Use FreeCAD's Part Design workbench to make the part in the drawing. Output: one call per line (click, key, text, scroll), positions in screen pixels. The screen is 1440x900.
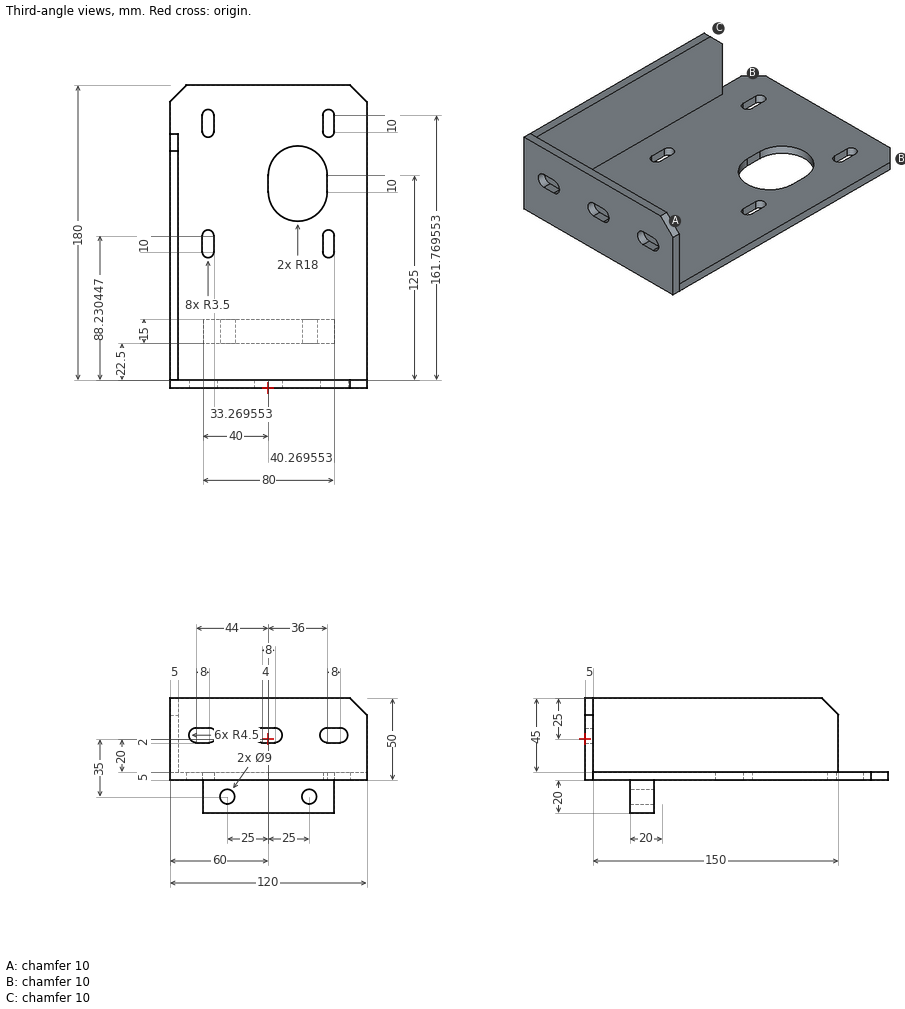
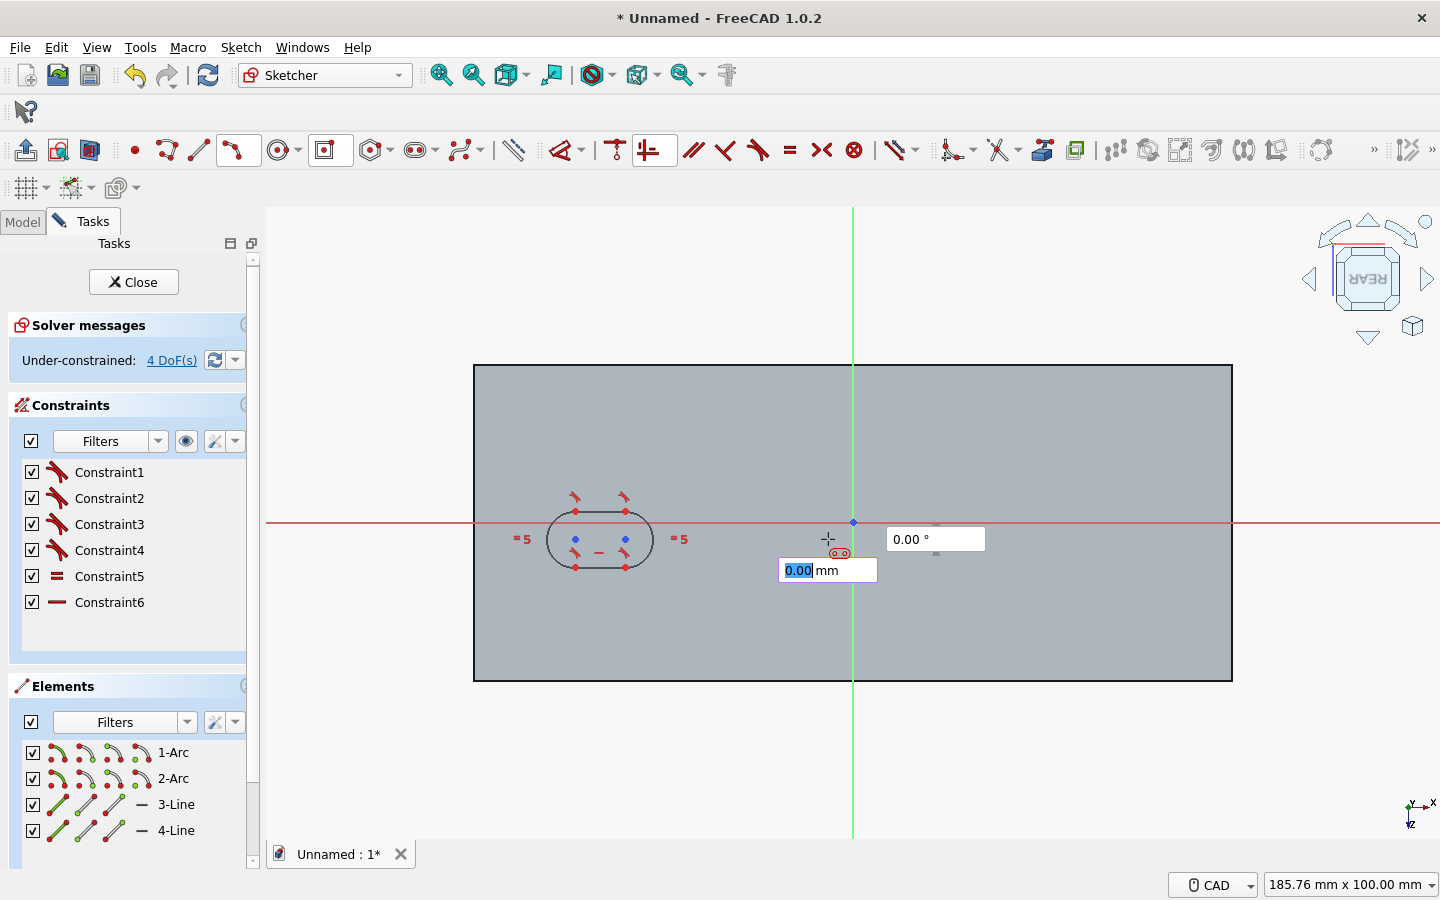
click(878, 539)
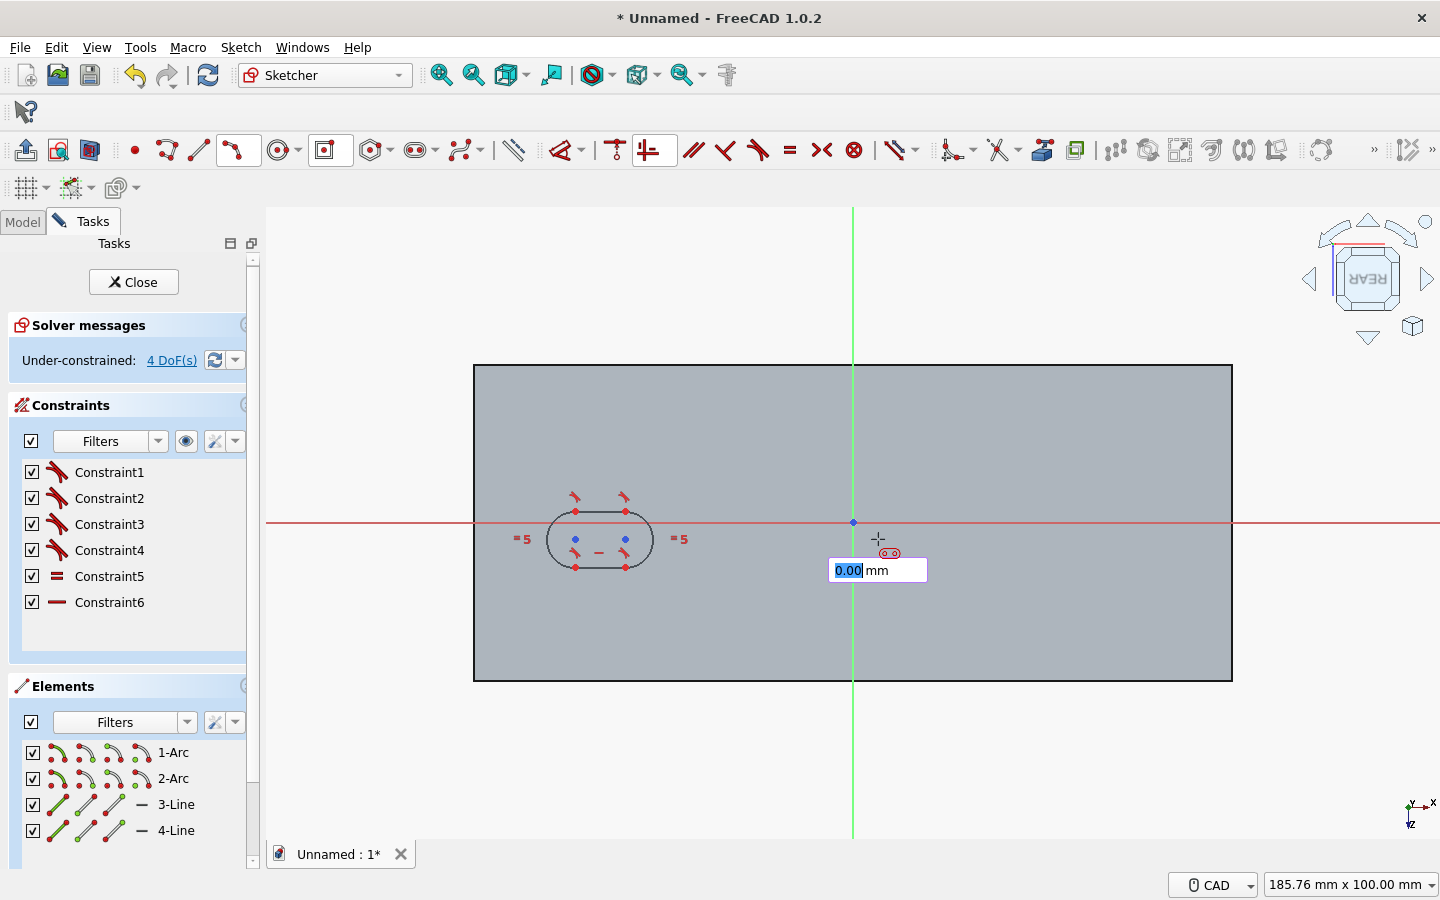
scroll(861, 510, up, 4)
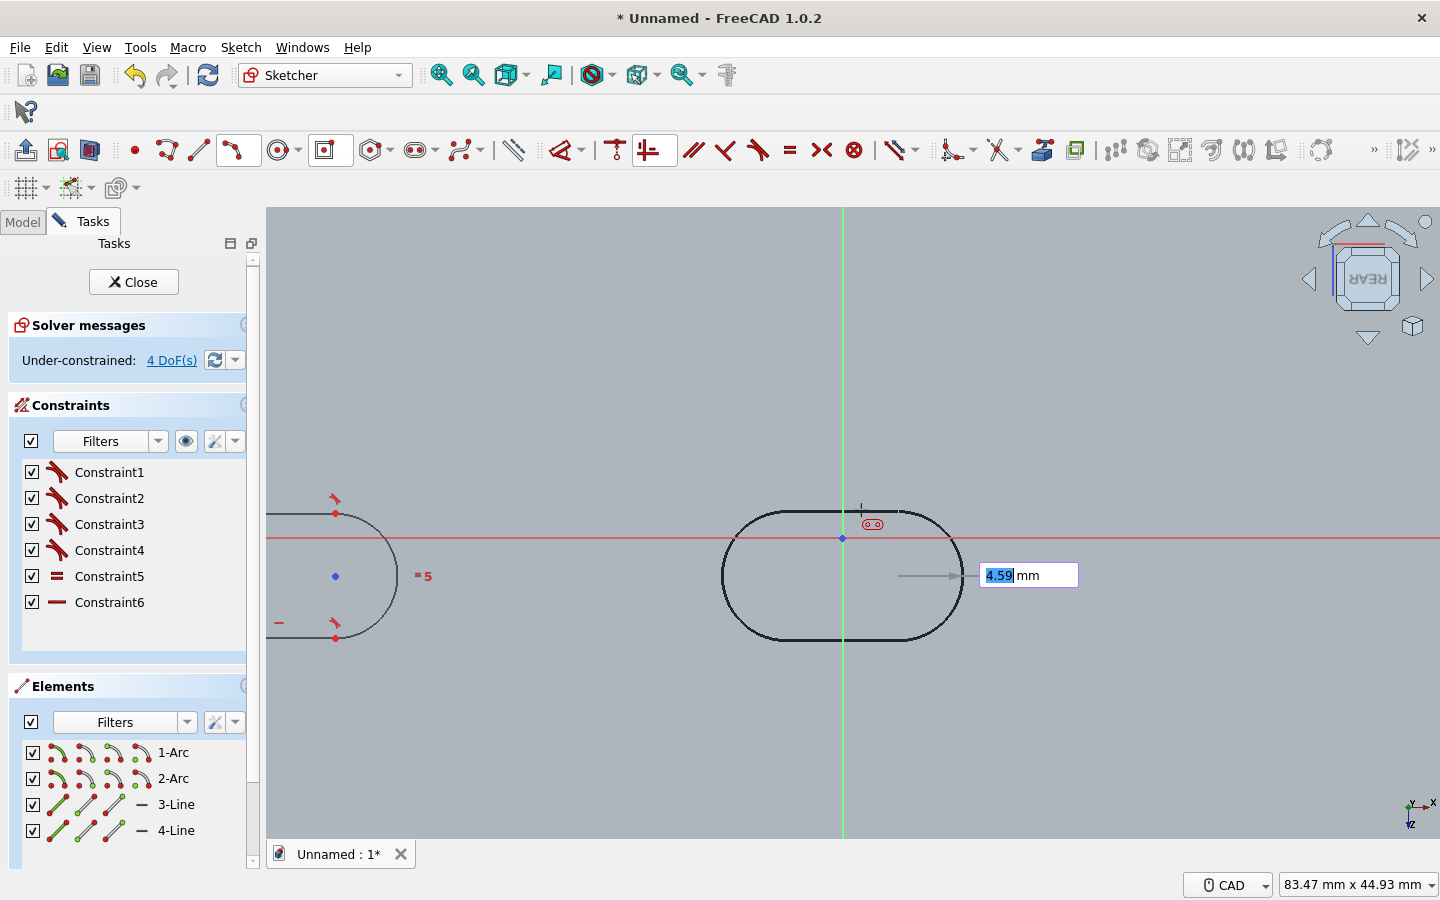
click(859, 510)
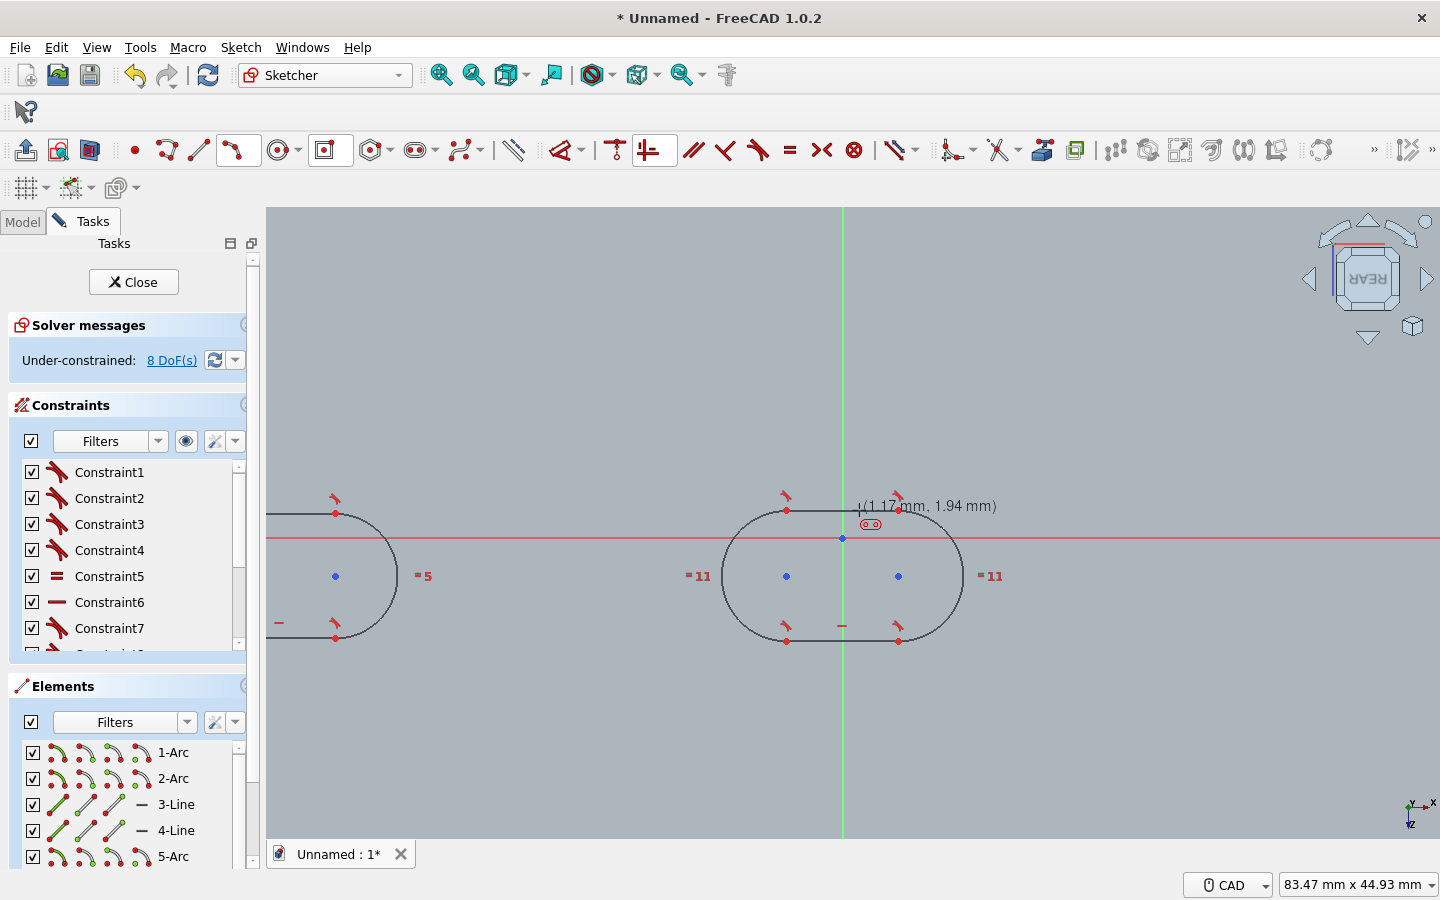
scroll(714, 462, down, 3)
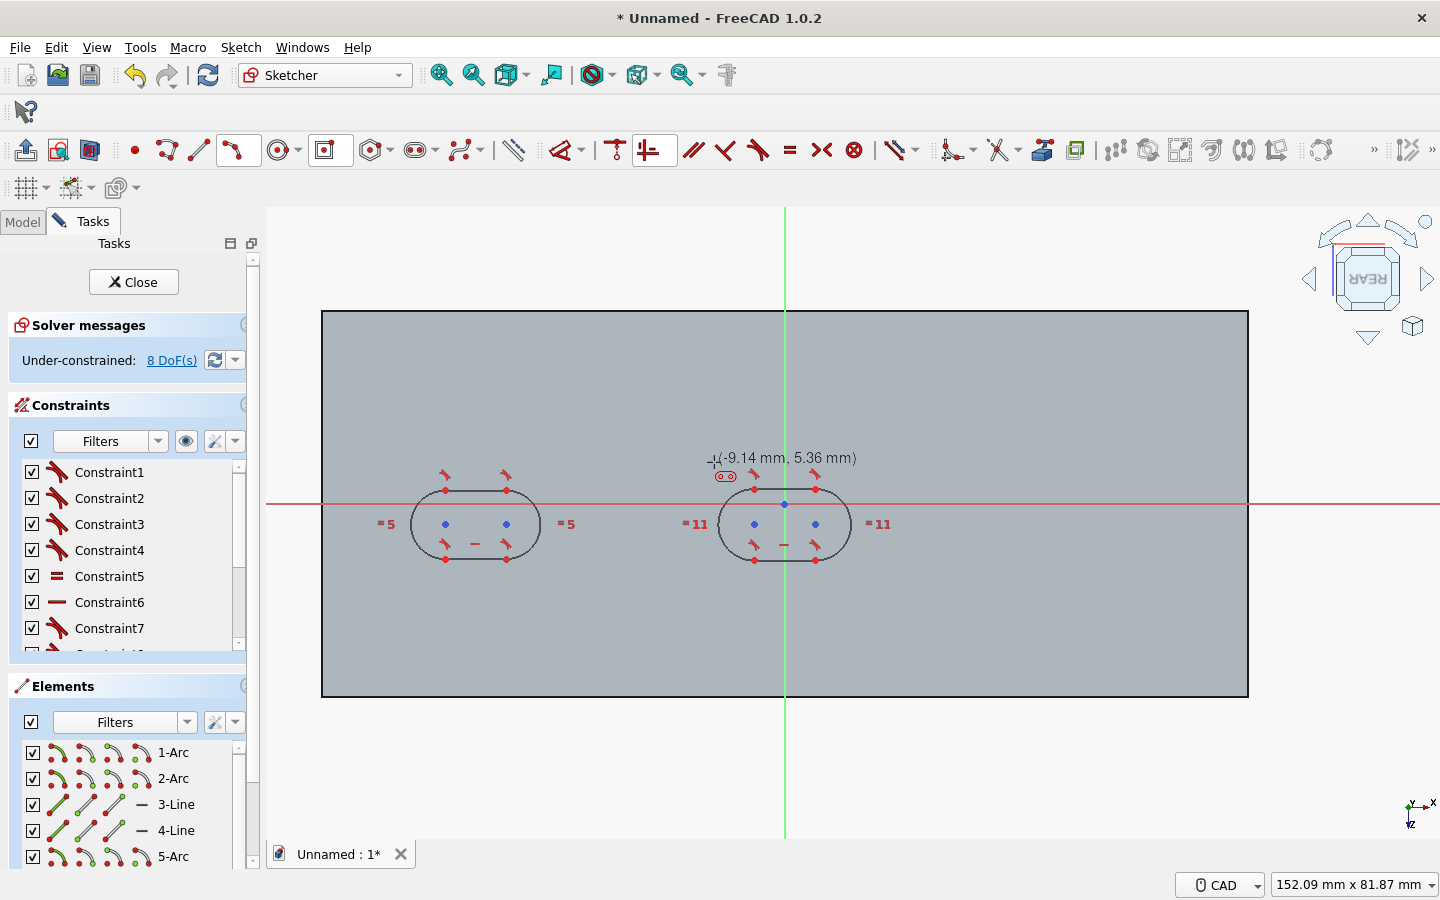
click(1063, 523)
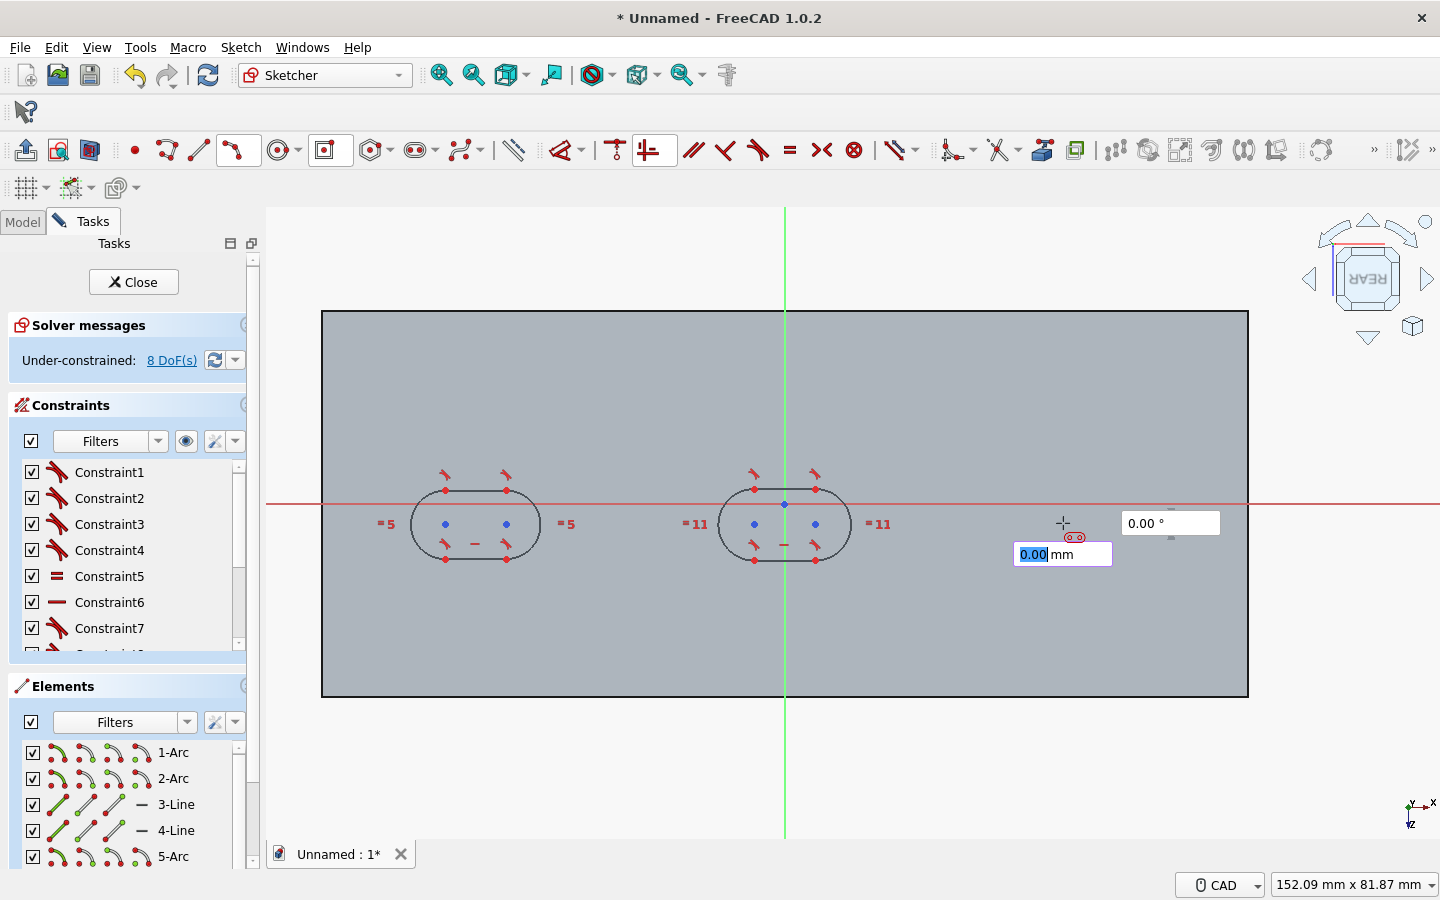
click(1124, 523)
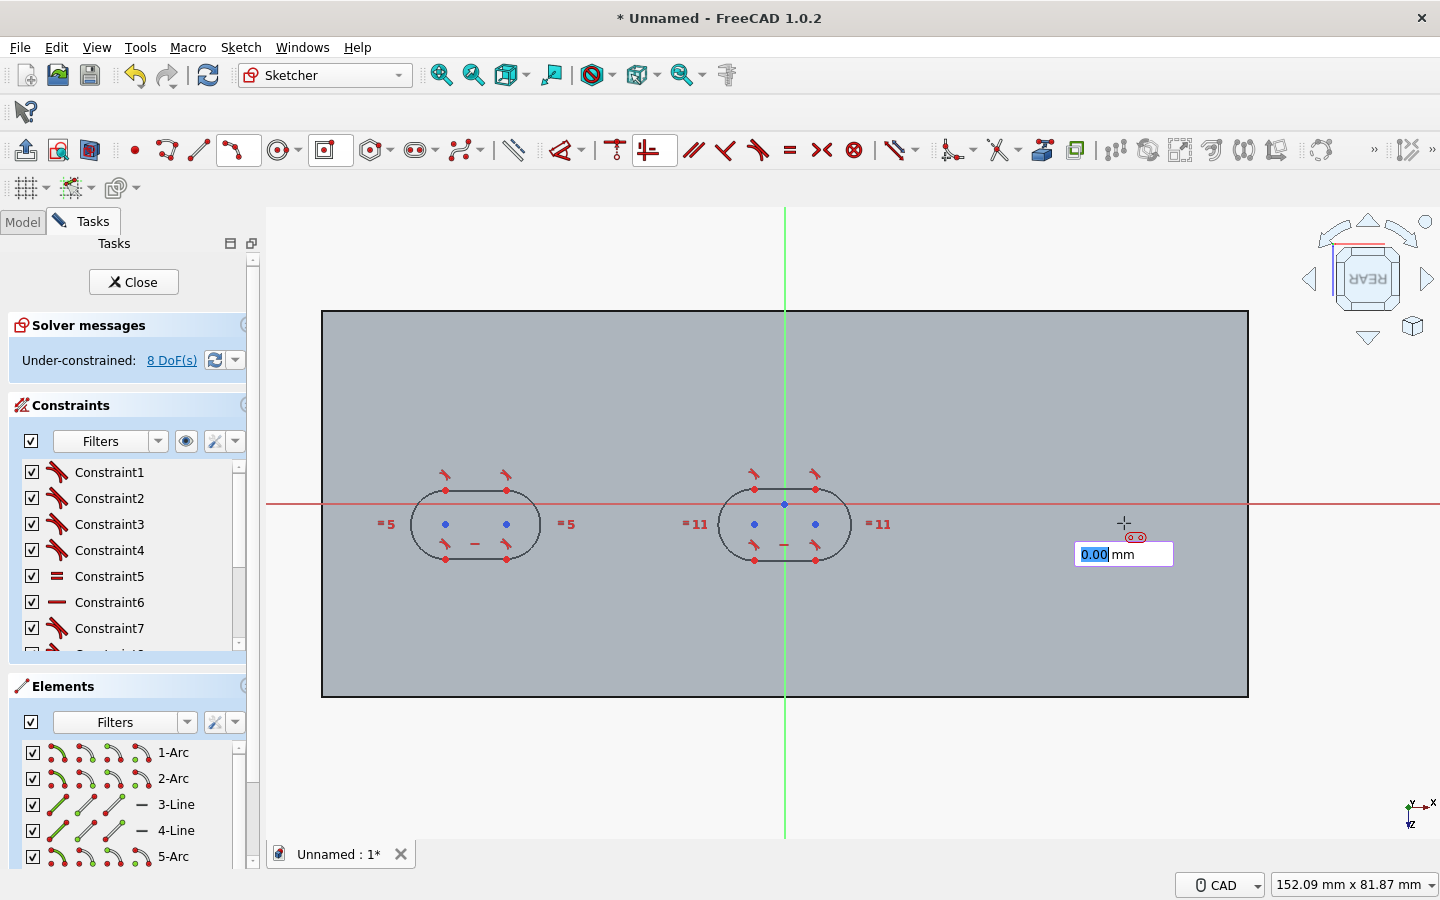
click(1094, 489)
key(Escape)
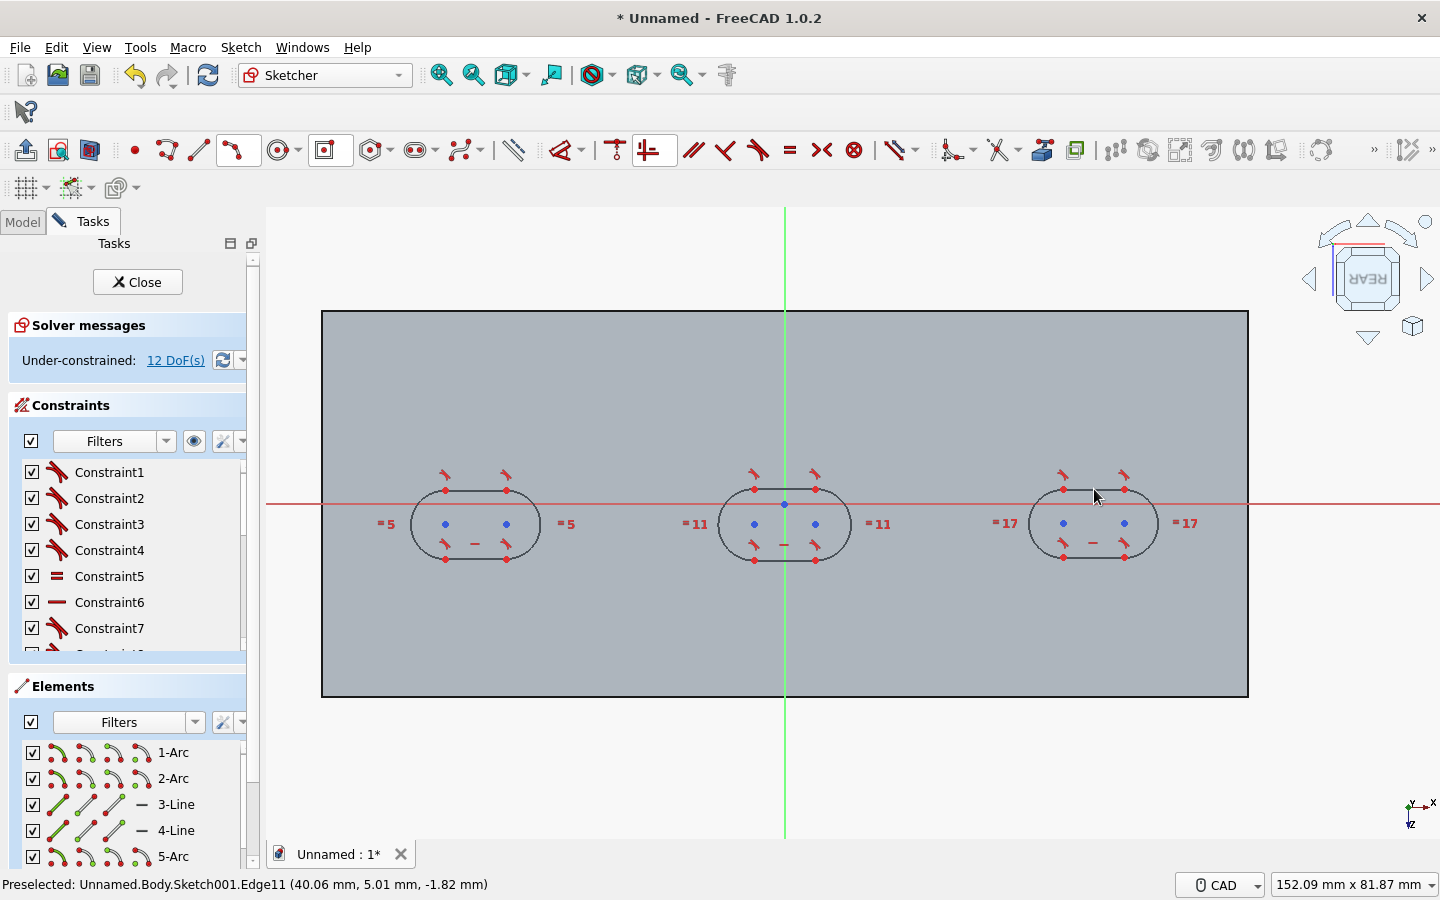
click(418, 505)